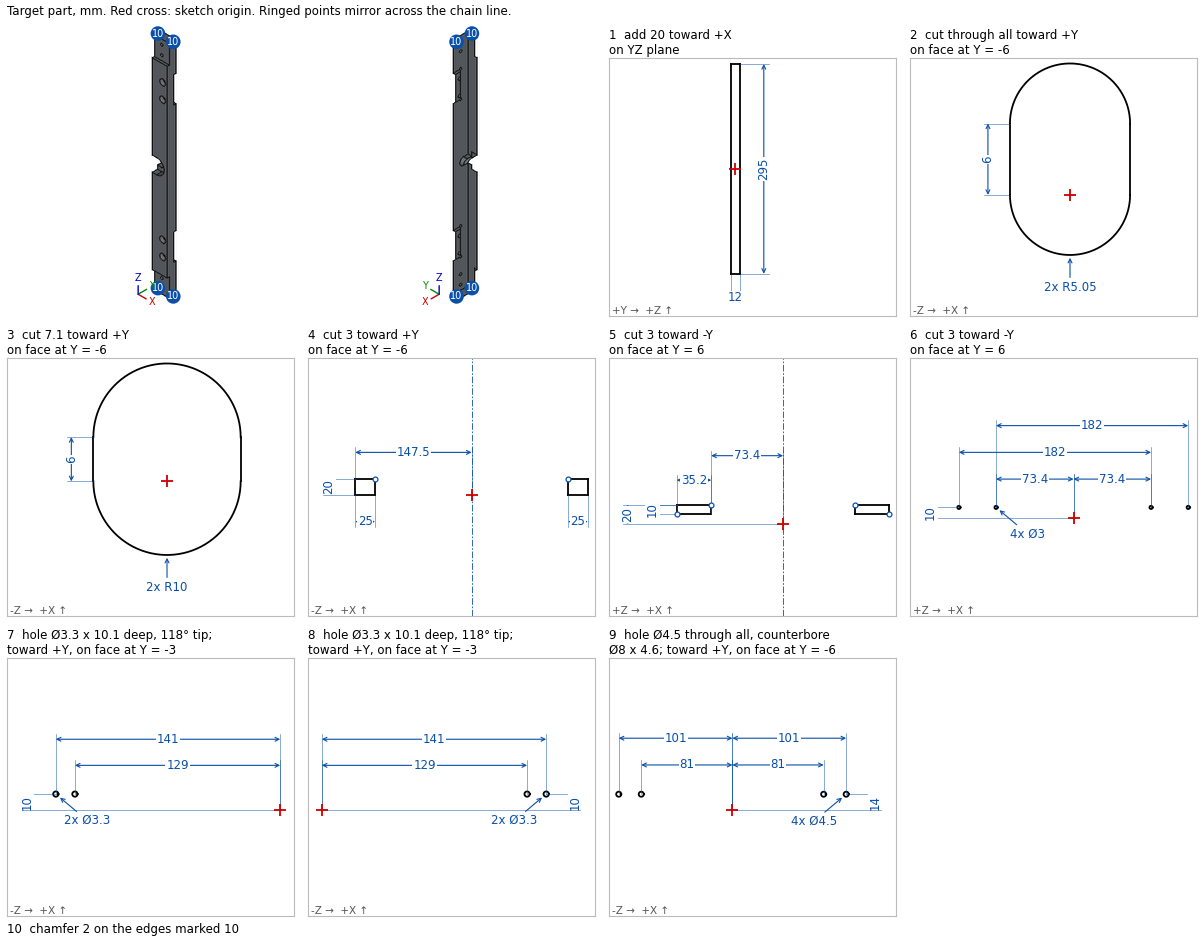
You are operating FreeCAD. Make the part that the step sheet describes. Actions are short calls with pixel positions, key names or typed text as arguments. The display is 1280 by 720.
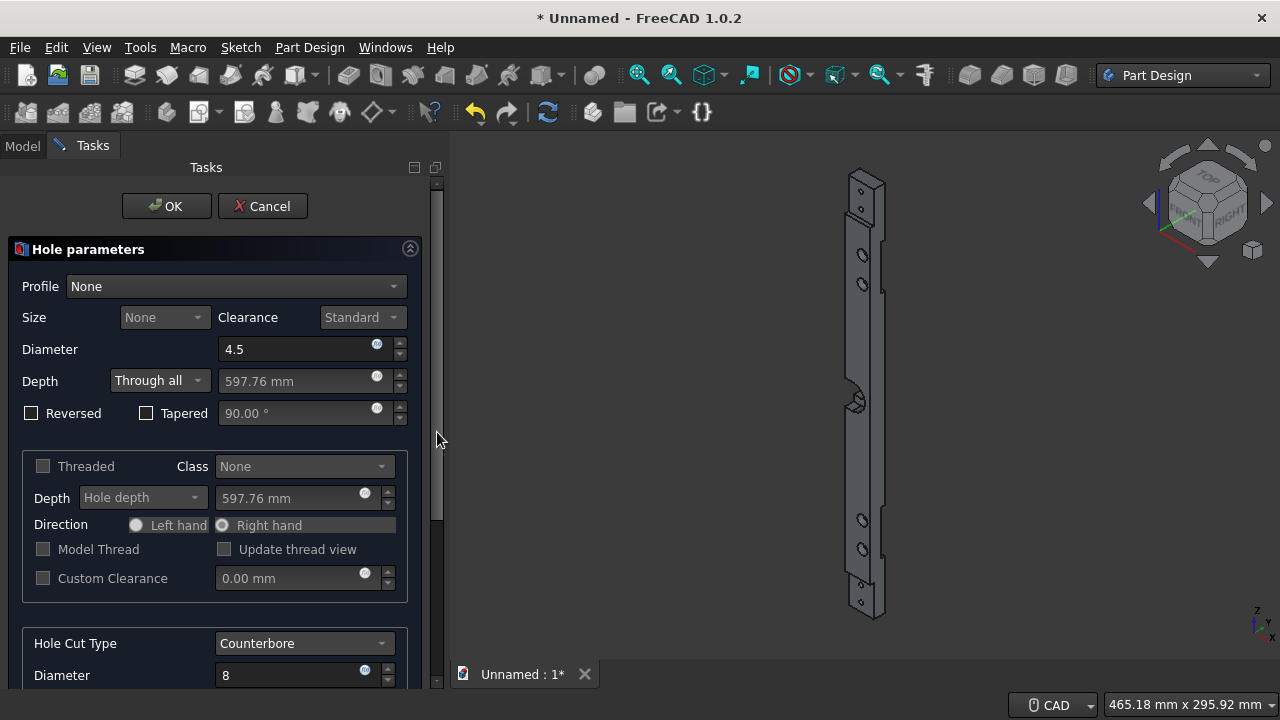
click(167, 206)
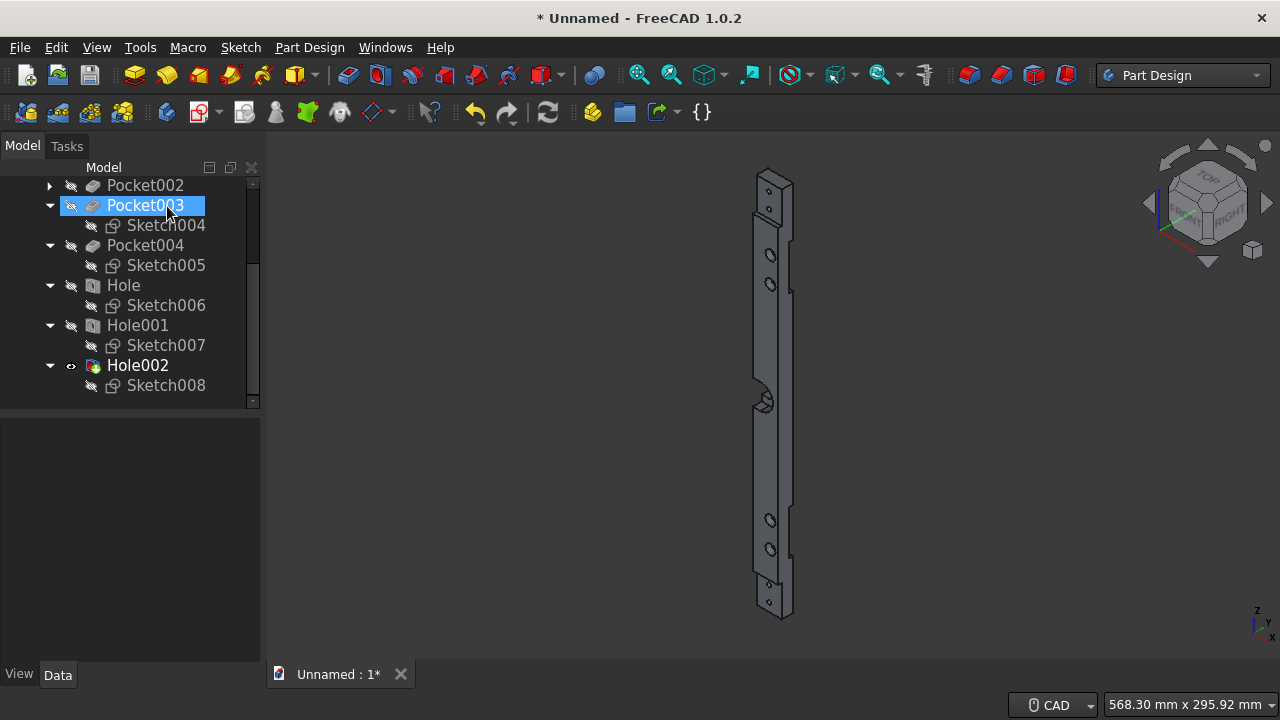
click(788, 185)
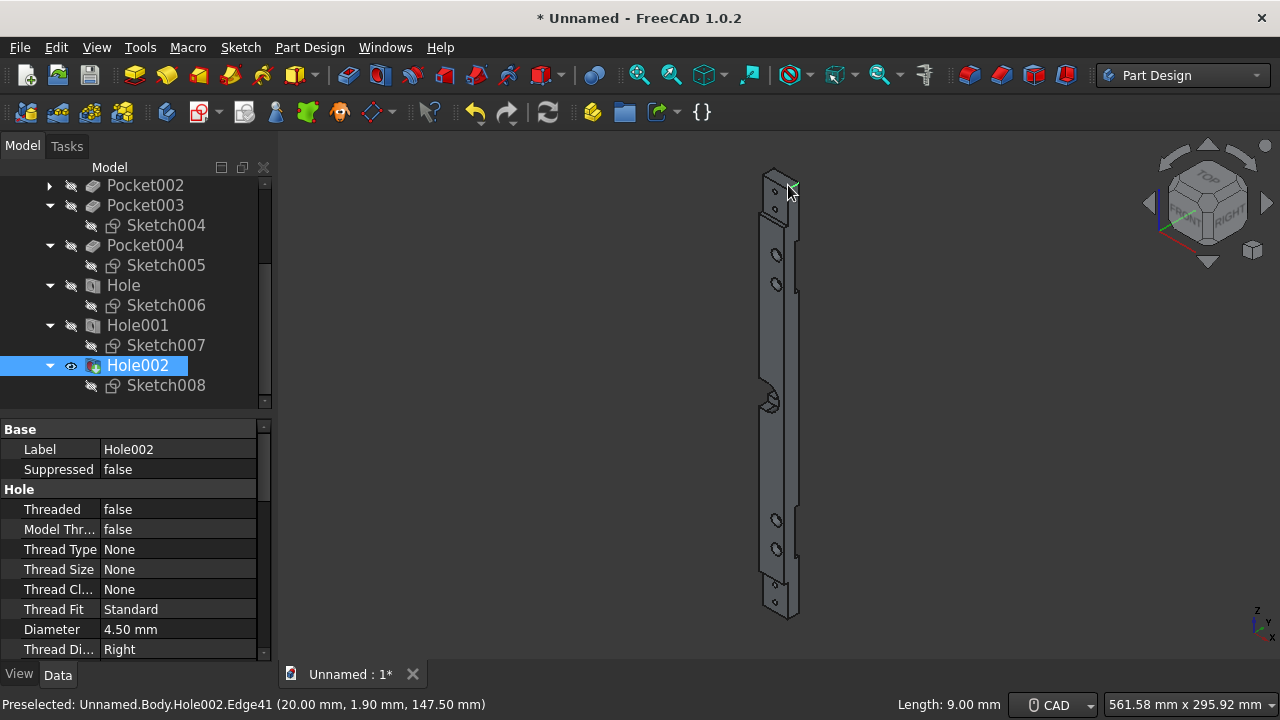
scroll(768, 171, up, 5)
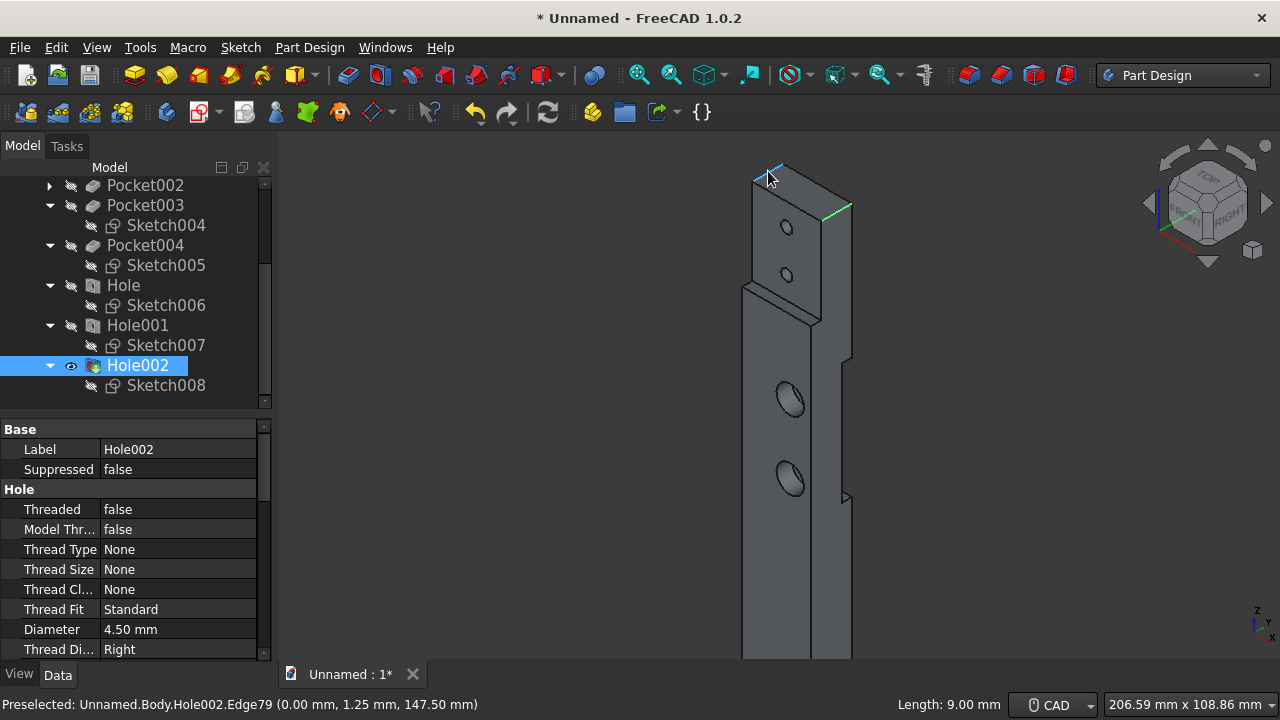
click(640, 76)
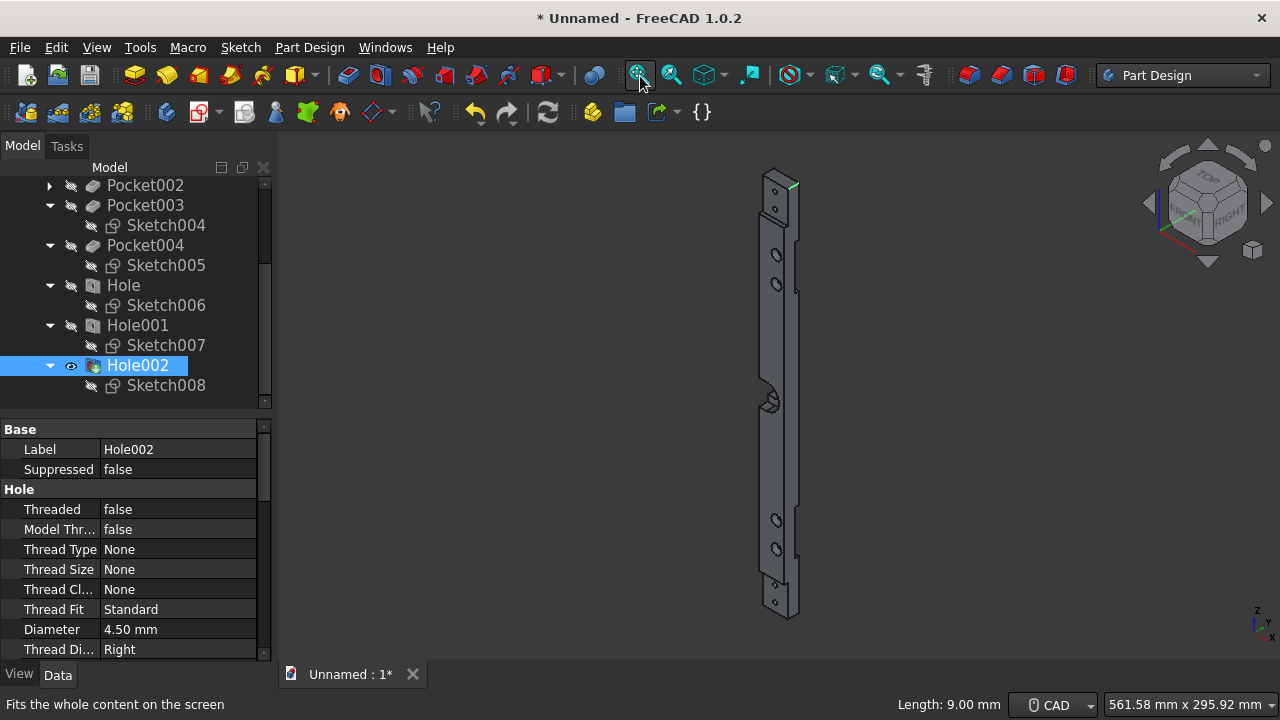
key(2)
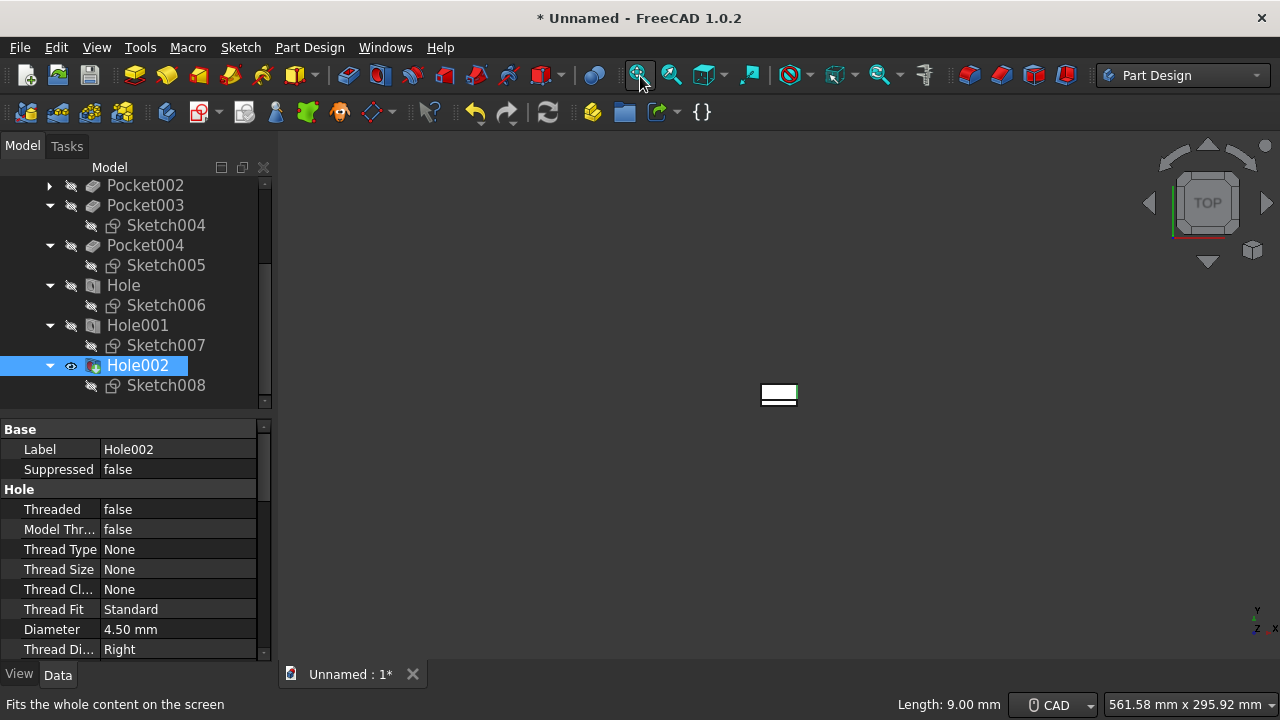
click(640, 76)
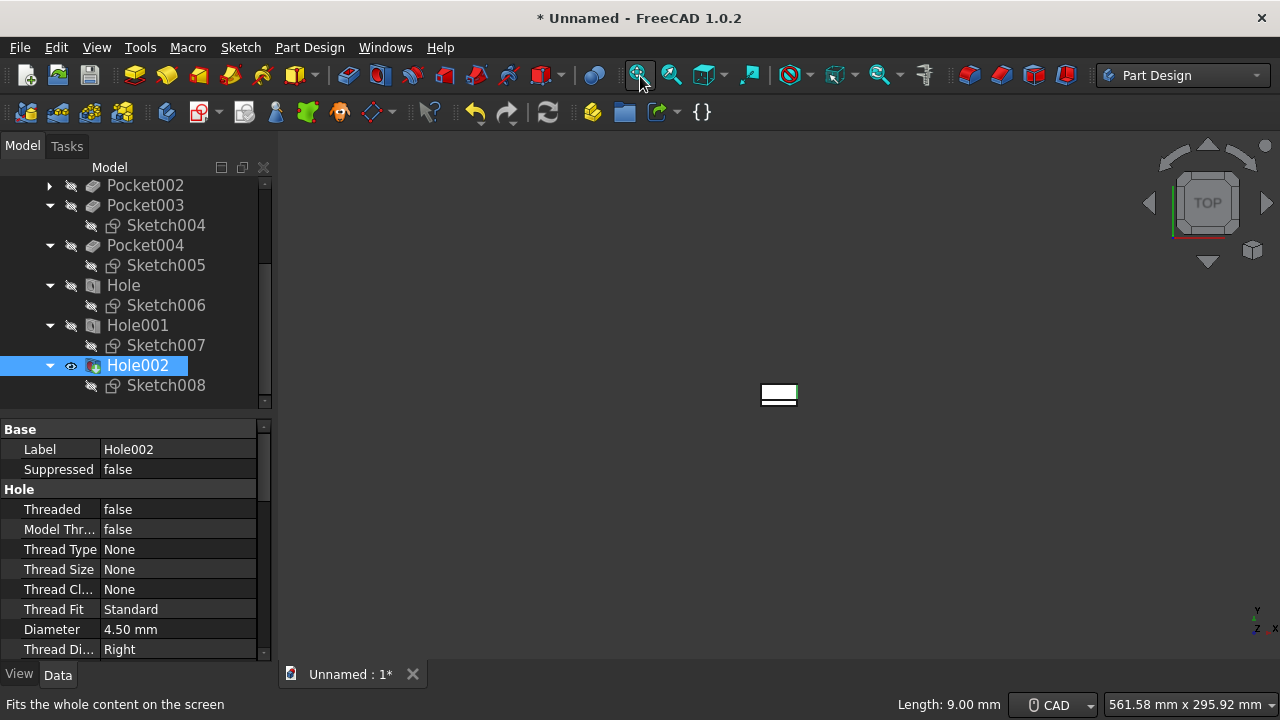
click(761, 391, ctrl)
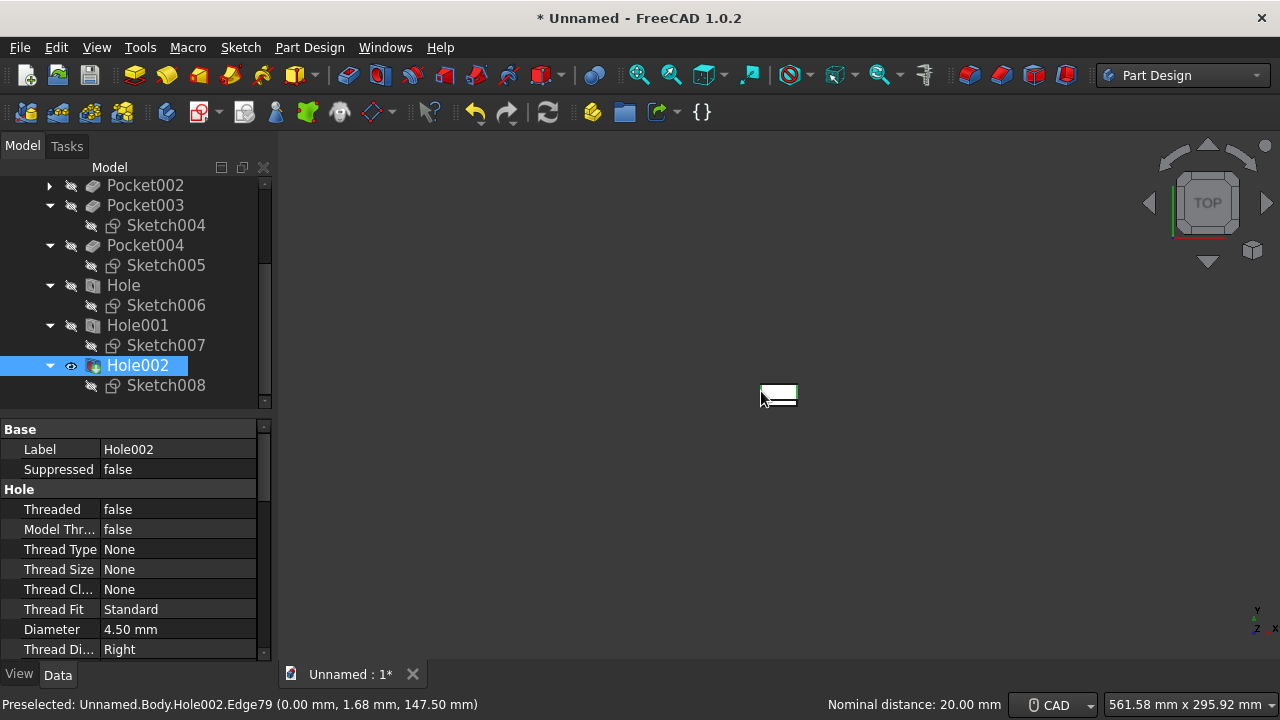
scroll(761, 391, up, 5)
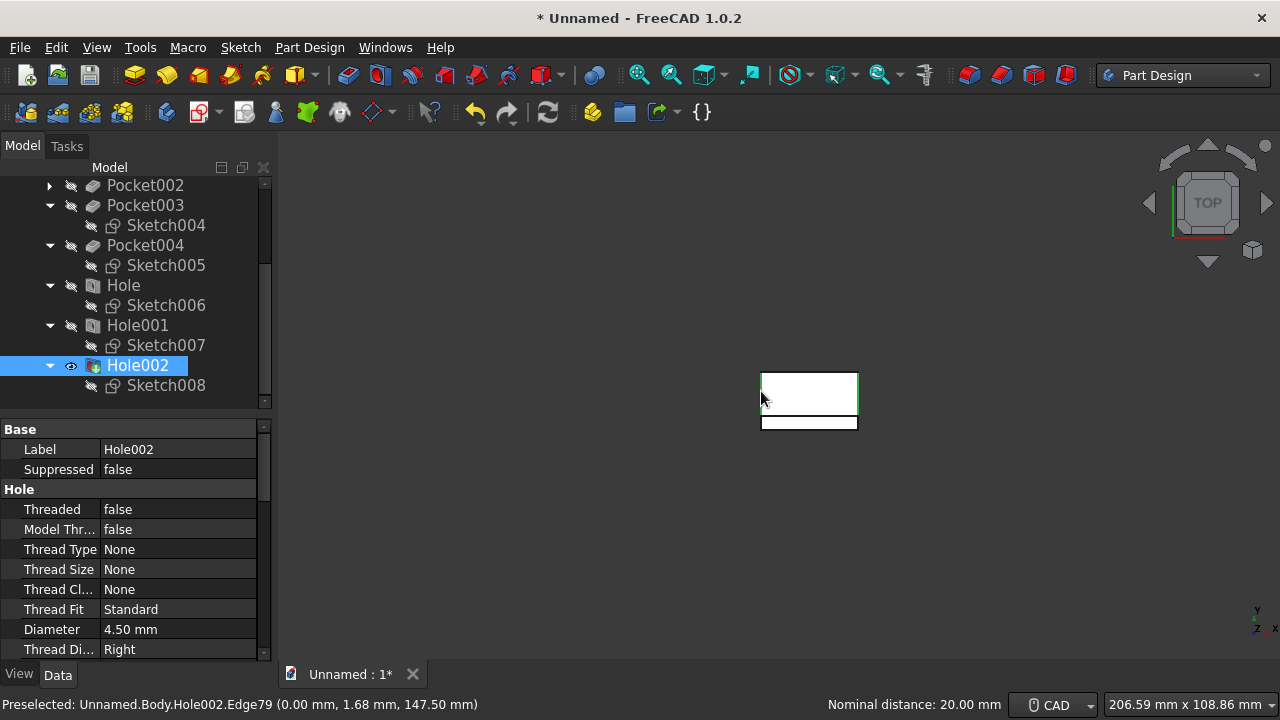
click(640, 76)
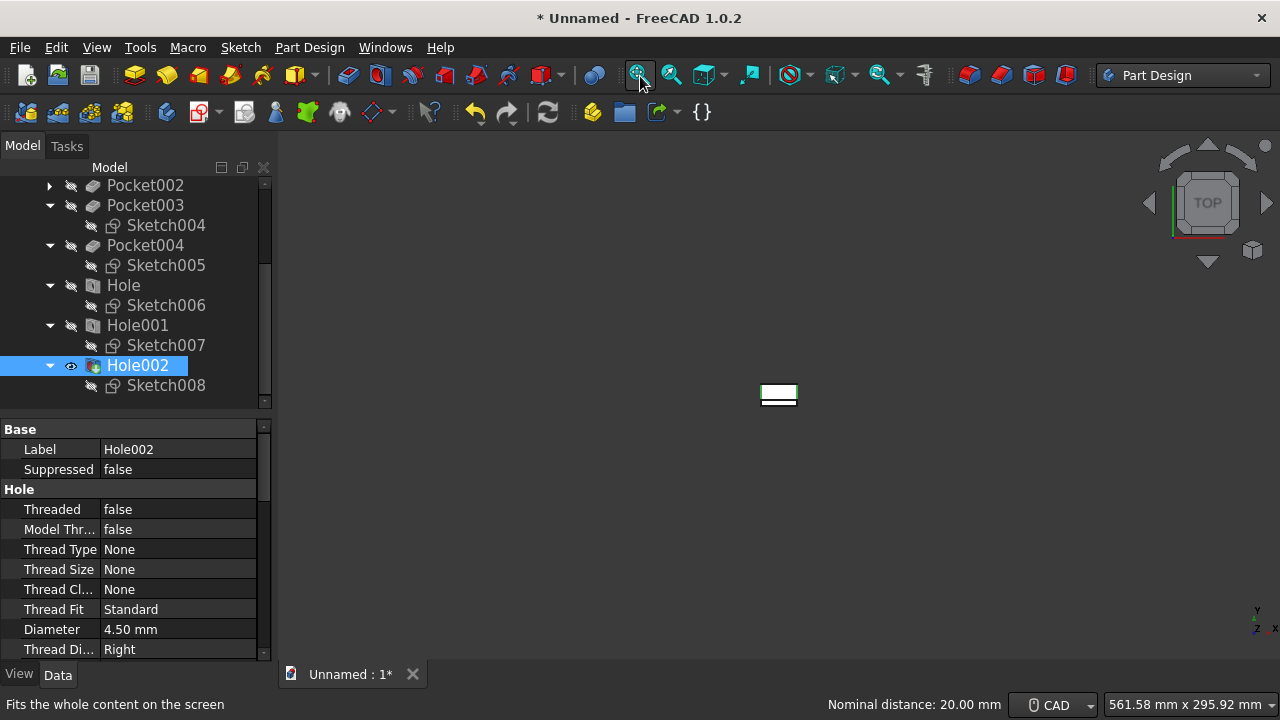
key(0)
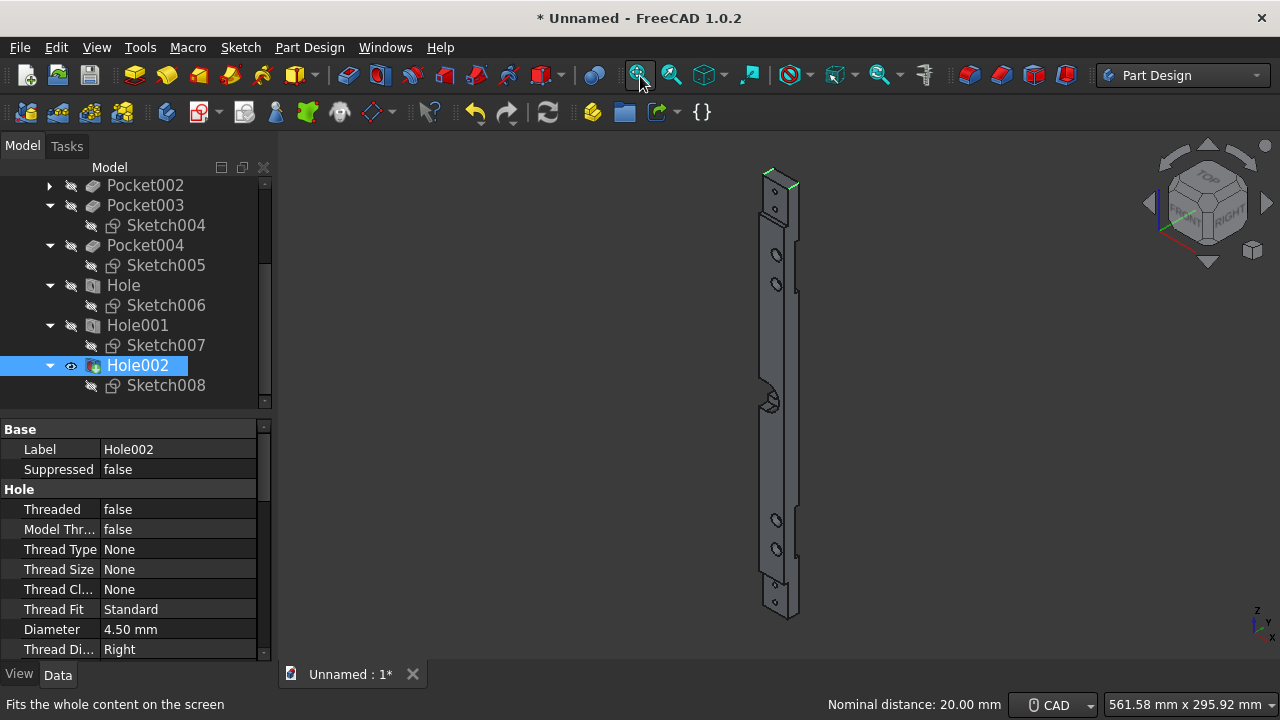
scroll(768, 601, up, 5)